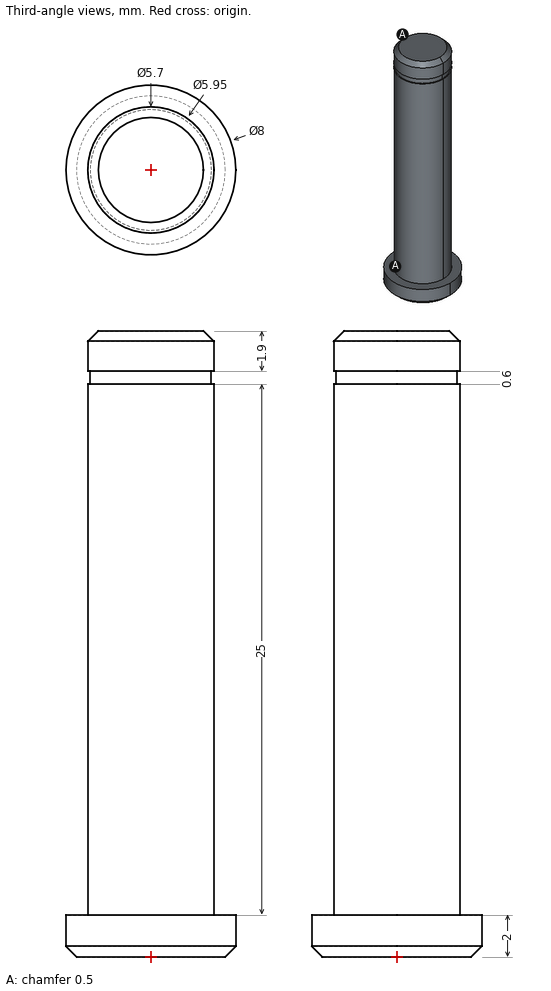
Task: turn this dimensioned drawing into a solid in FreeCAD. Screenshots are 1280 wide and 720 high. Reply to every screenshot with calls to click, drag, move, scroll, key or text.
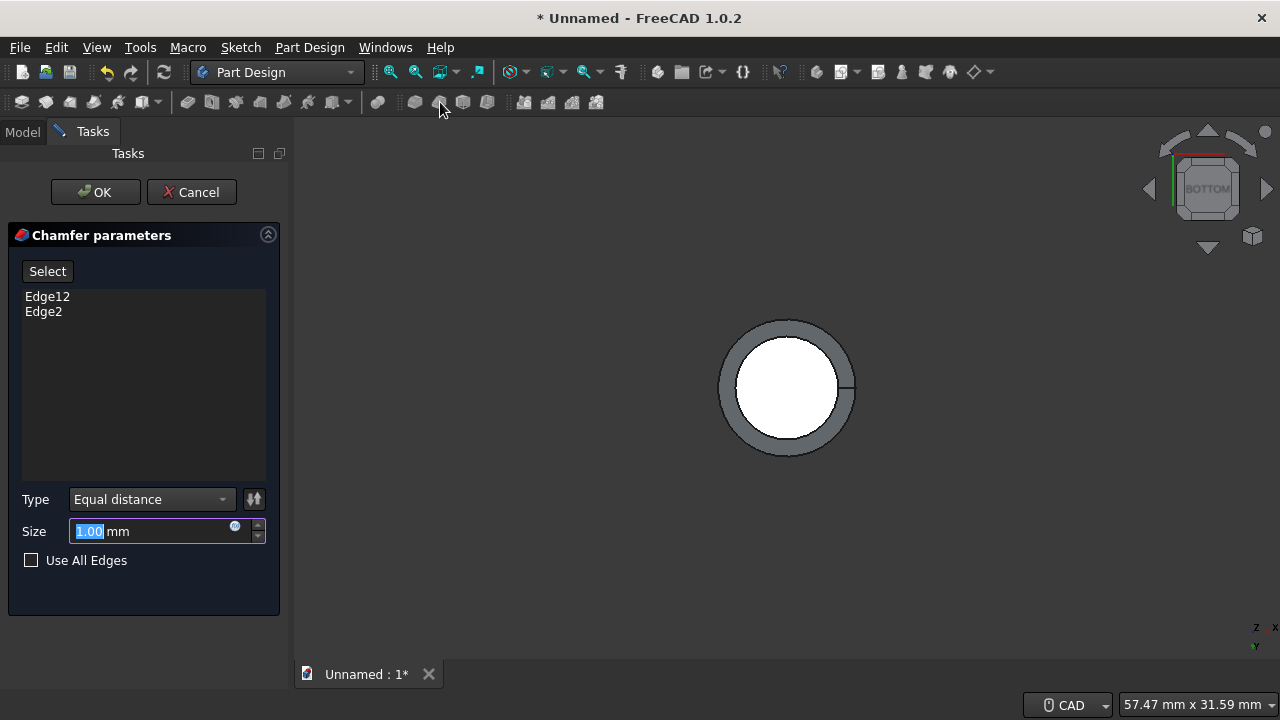
text(0.5)
key(Tab)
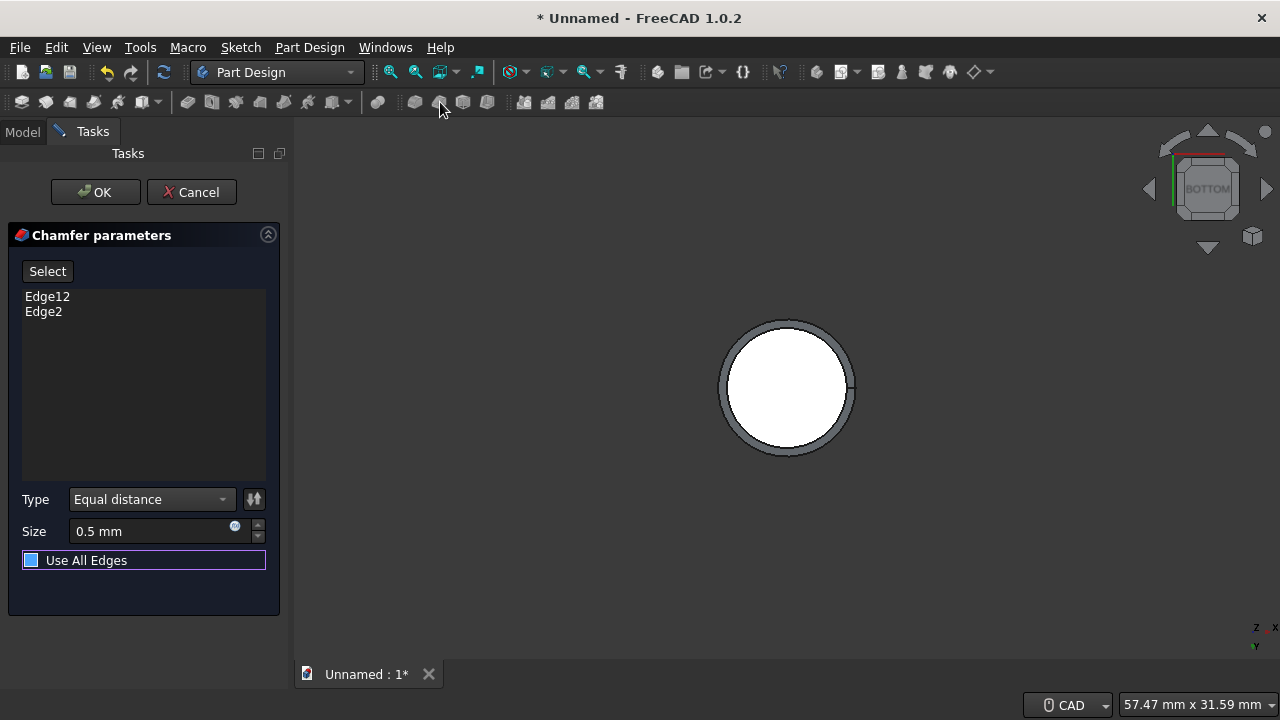
click(96, 192)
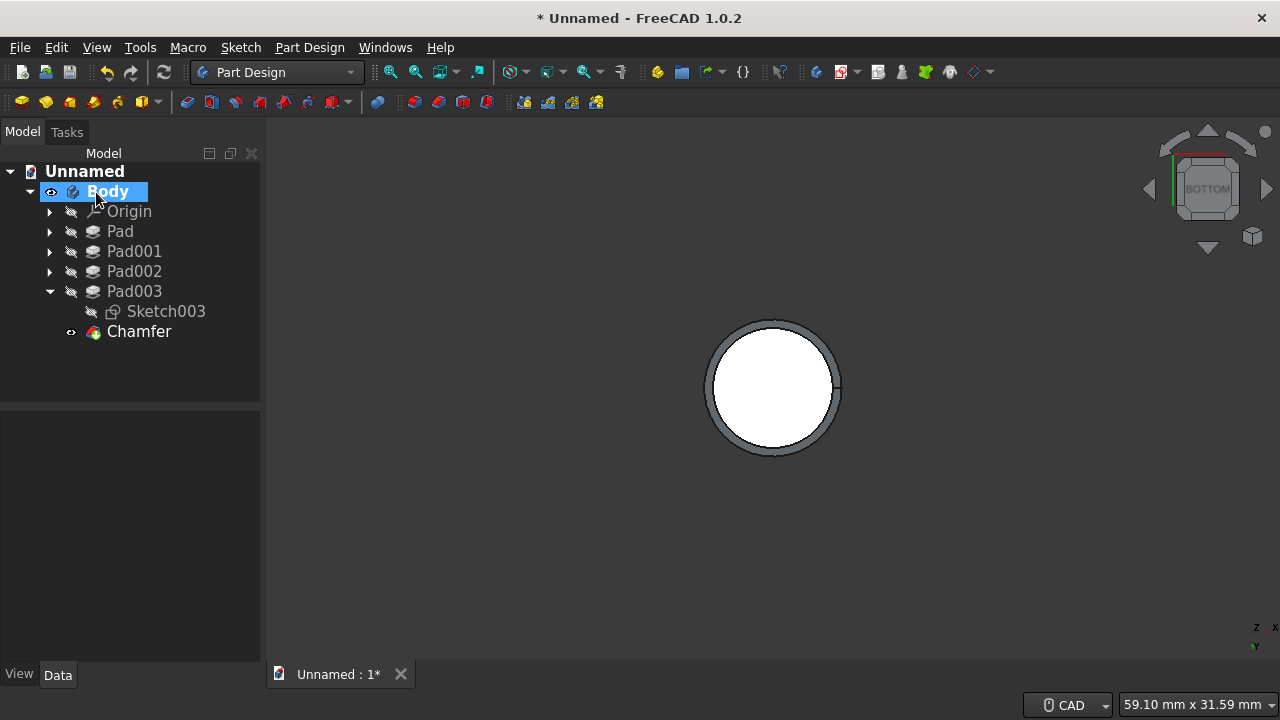
key(0)